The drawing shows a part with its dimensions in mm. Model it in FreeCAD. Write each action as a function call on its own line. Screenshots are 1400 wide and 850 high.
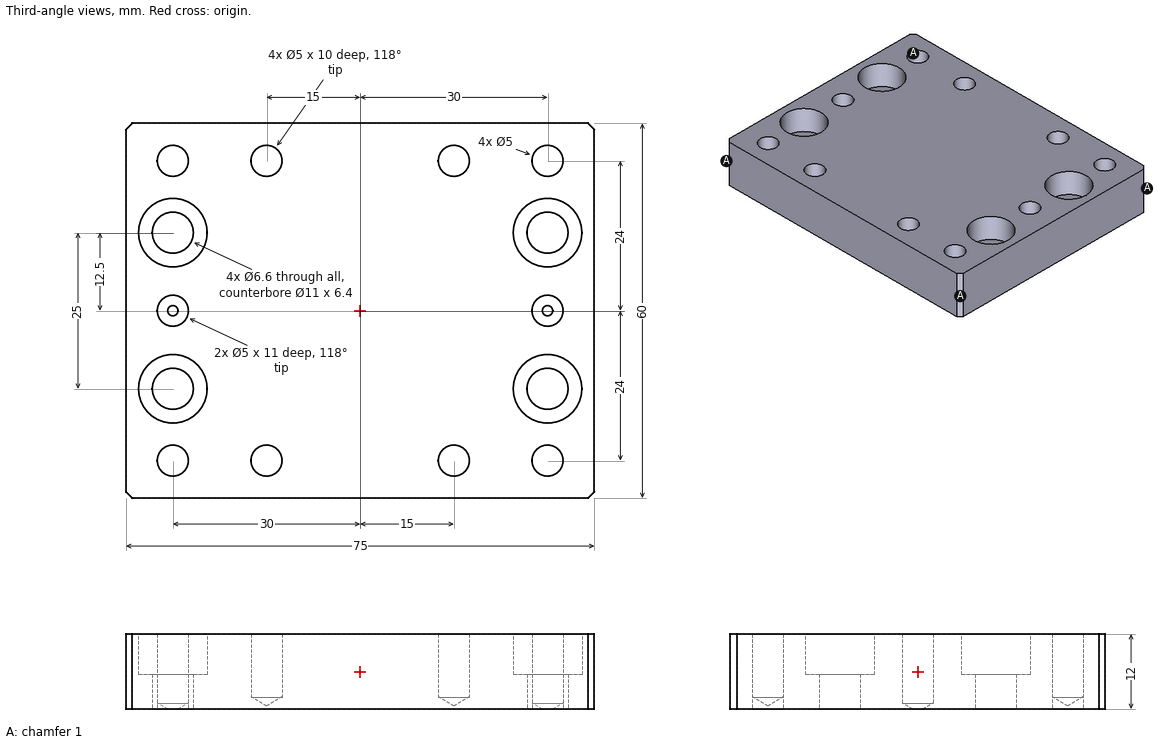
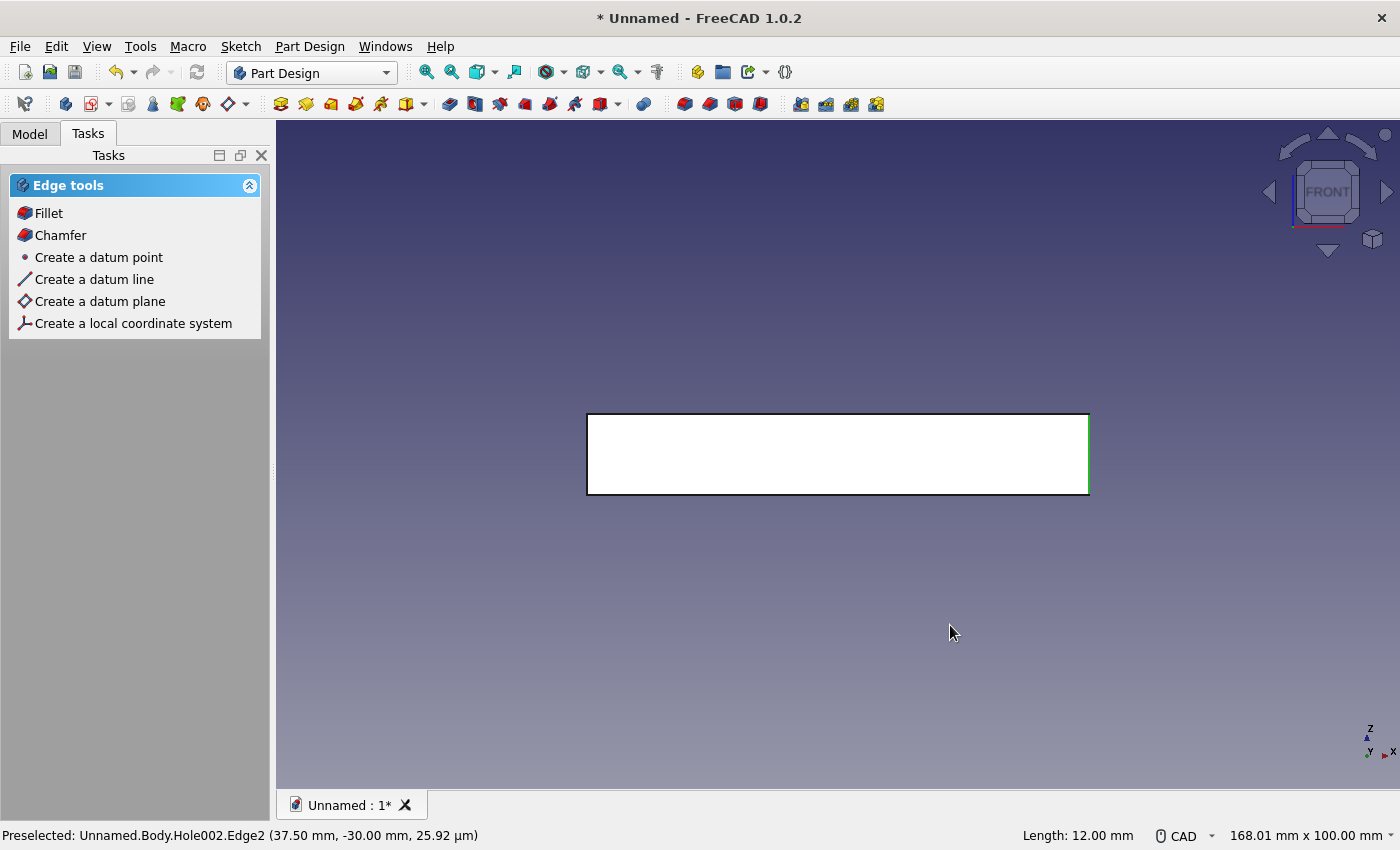
key(v)
key(f)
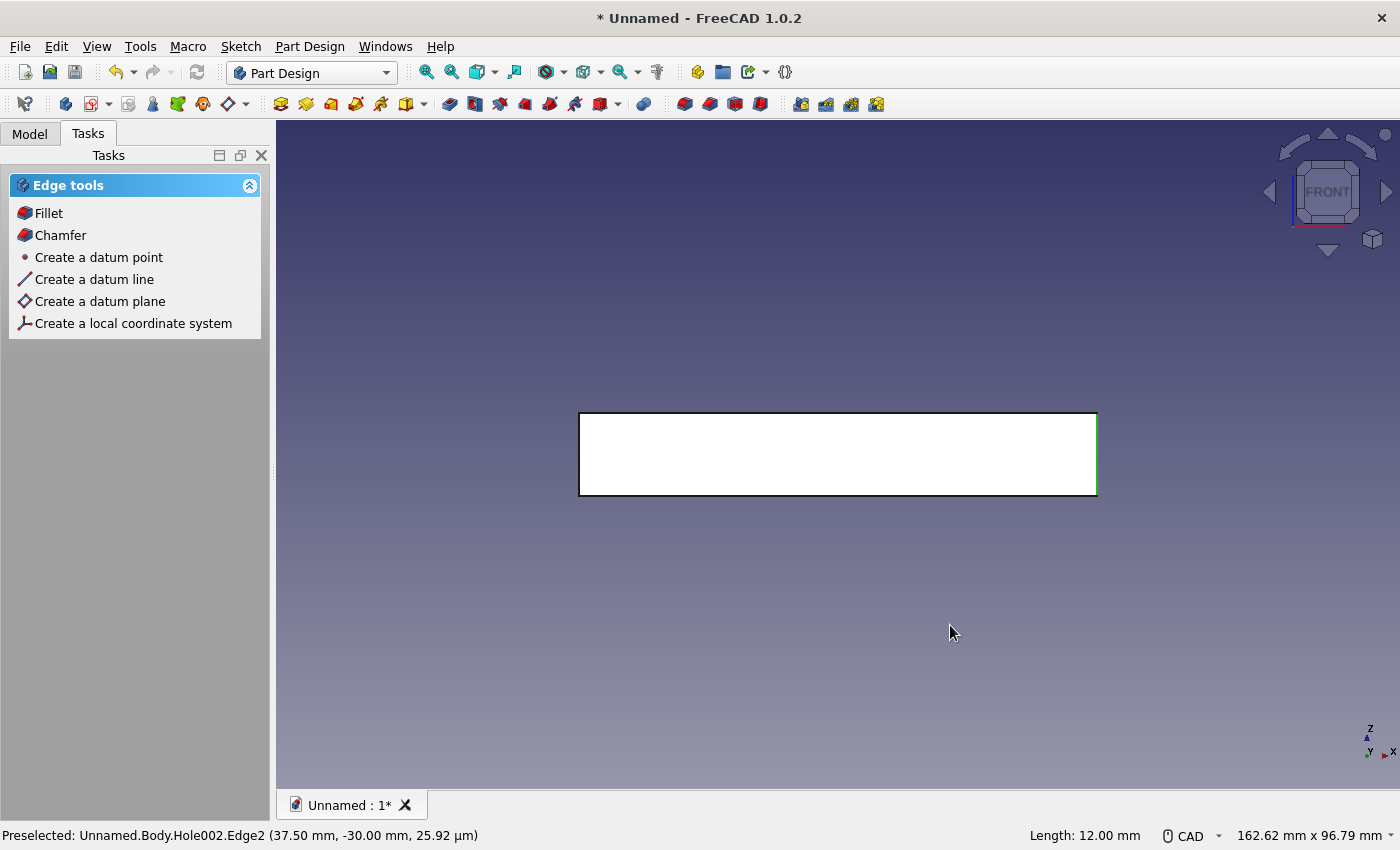
click(579, 454, ctrl)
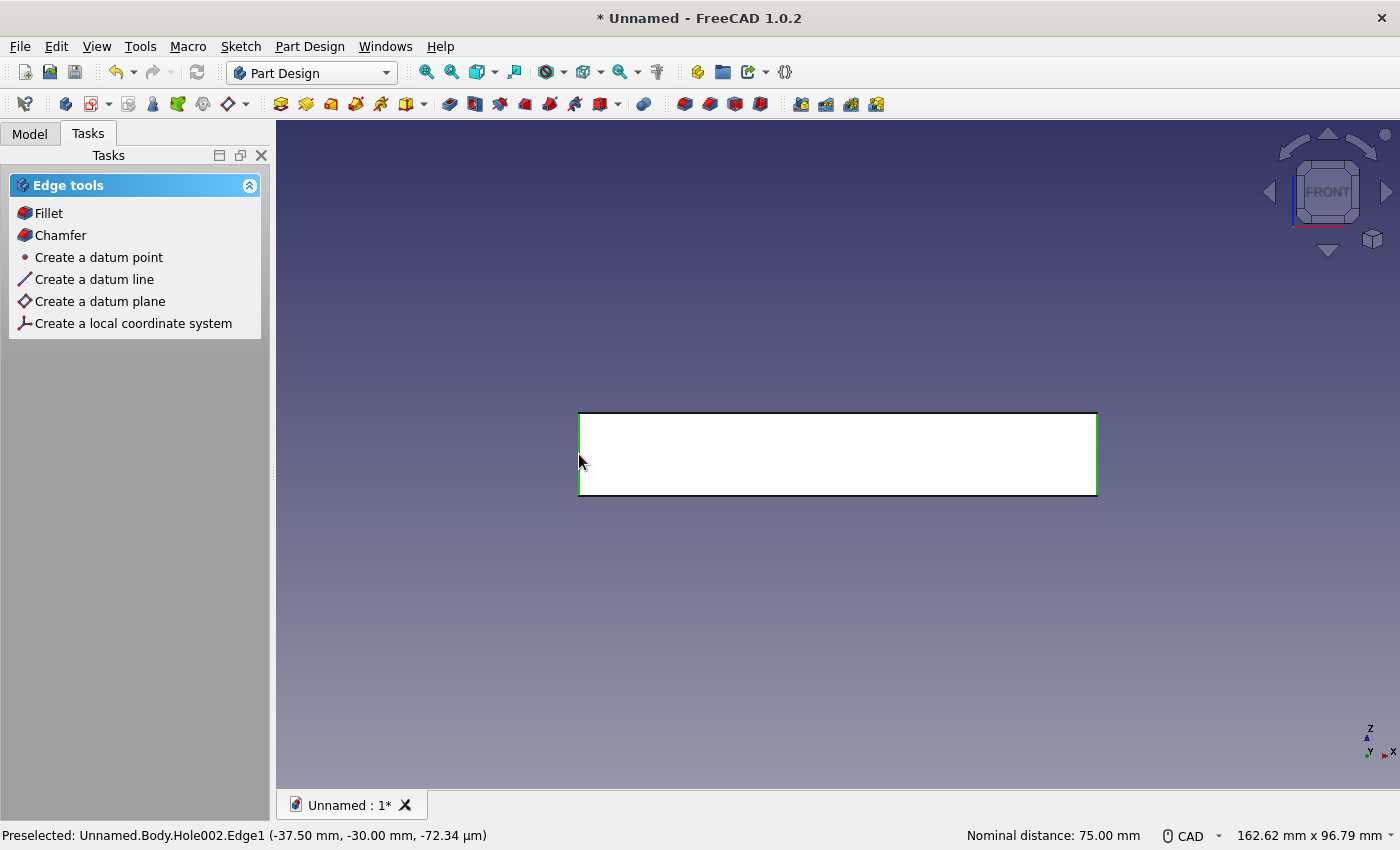
key(3)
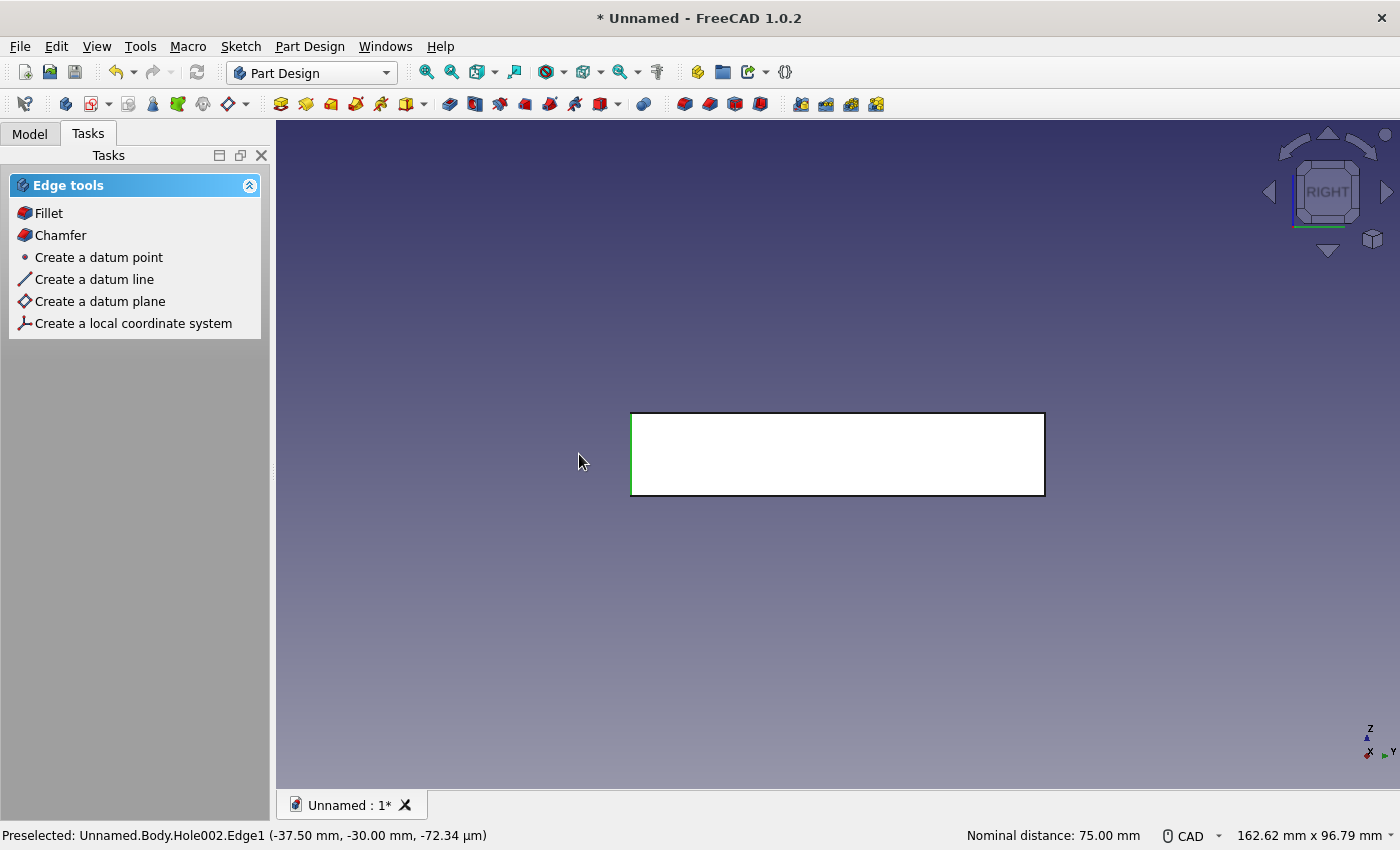
key(v)
key(f)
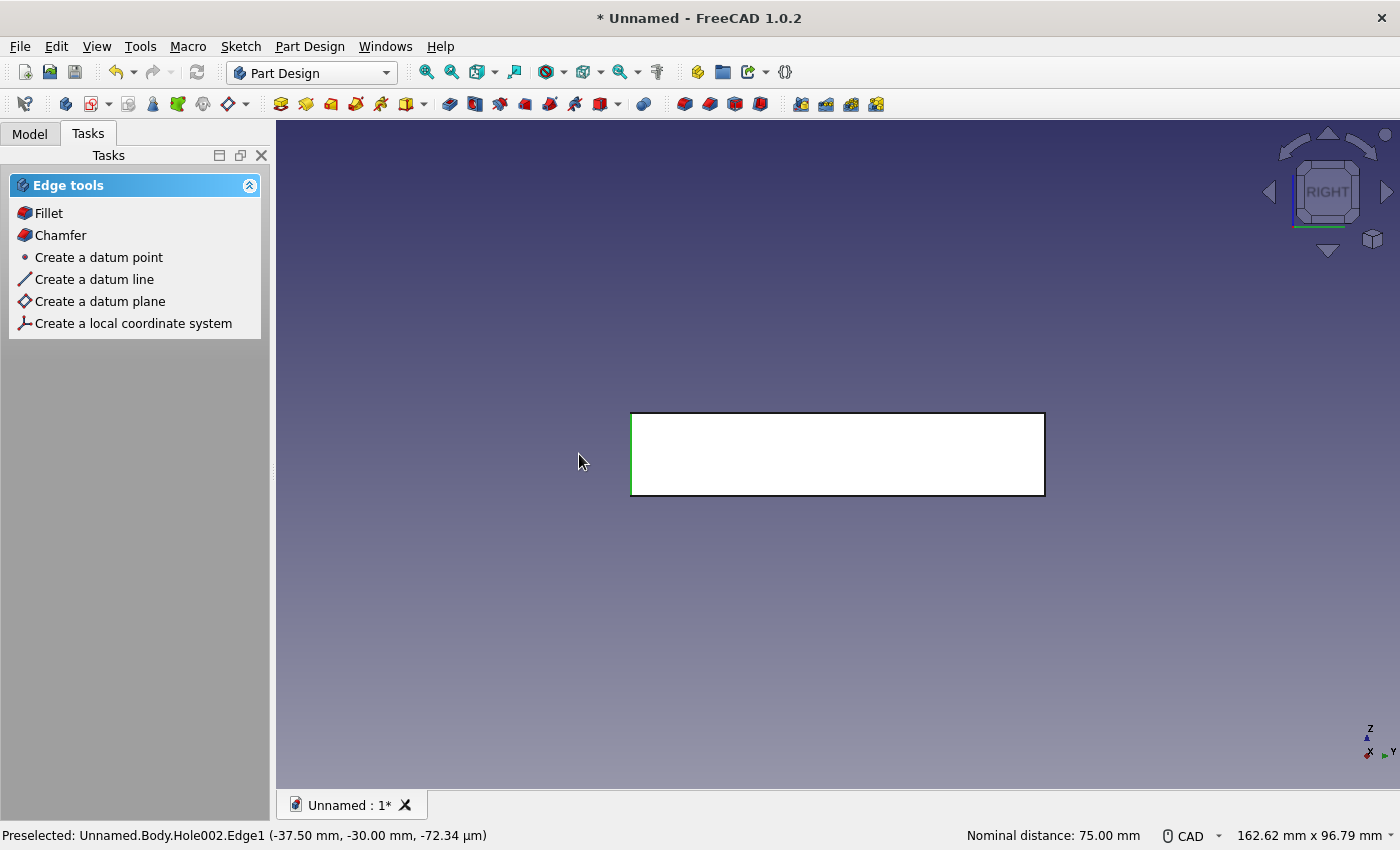
click(1045, 453, ctrl)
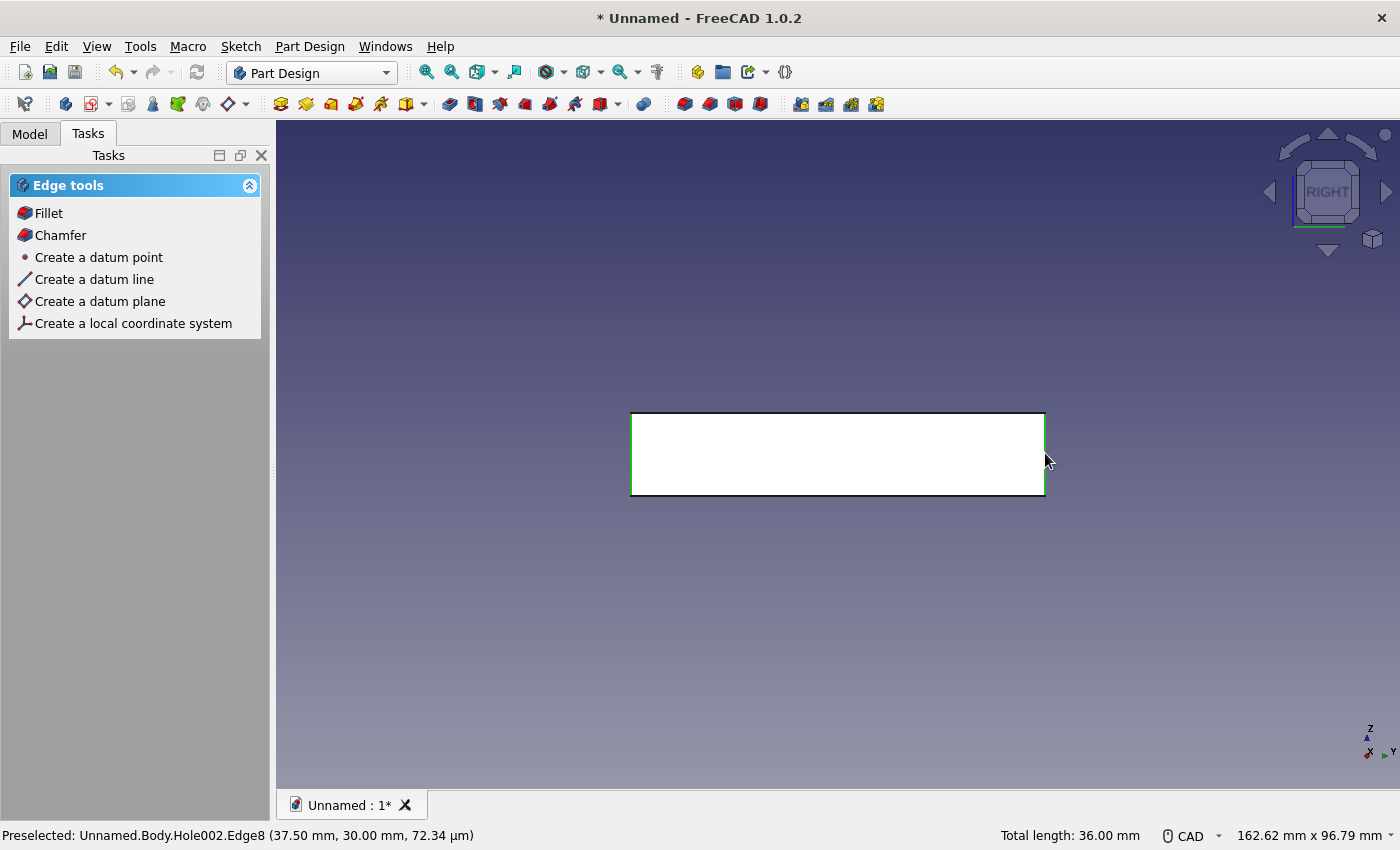
key(5)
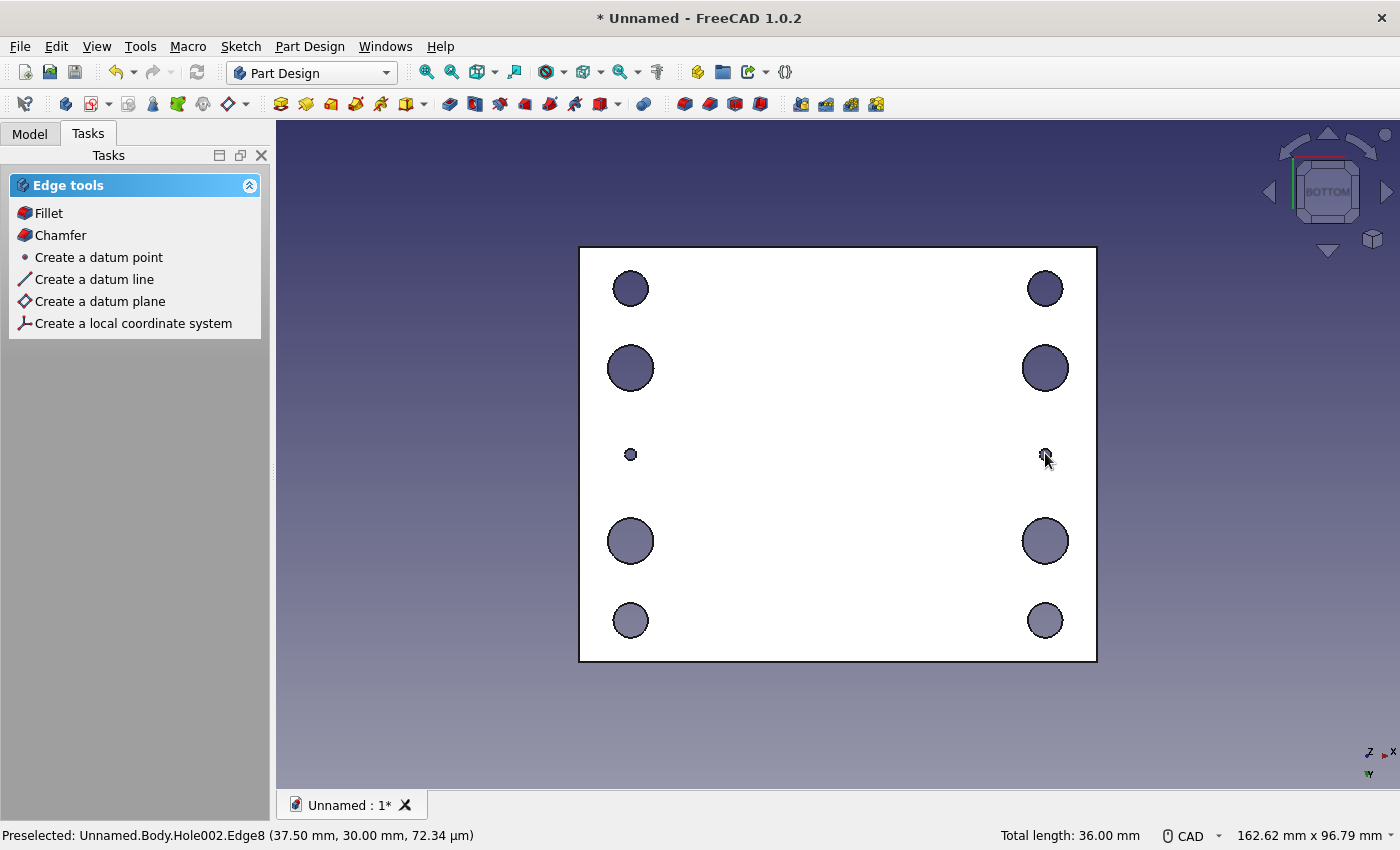
key(4)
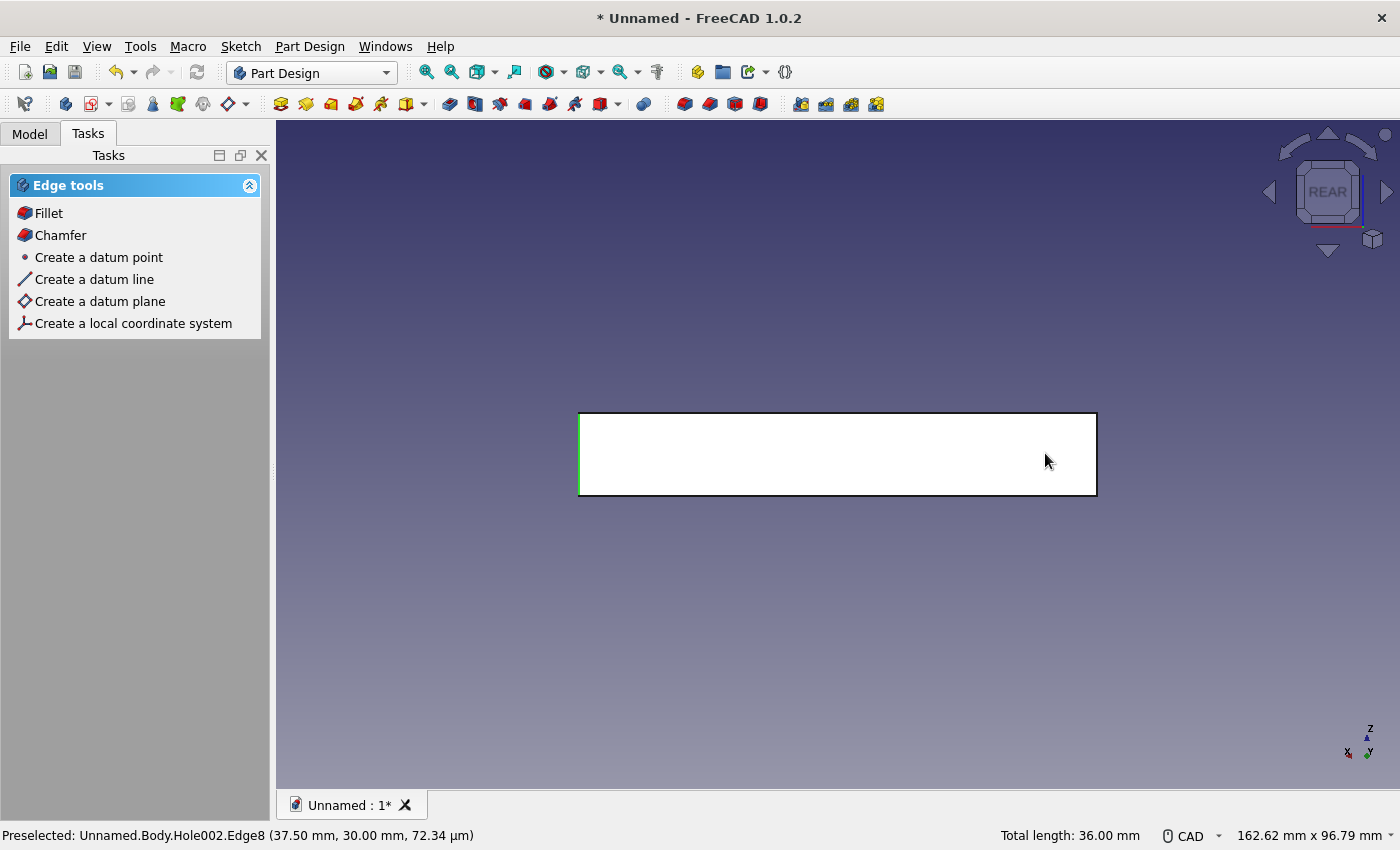
click(1097, 454, ctrl)